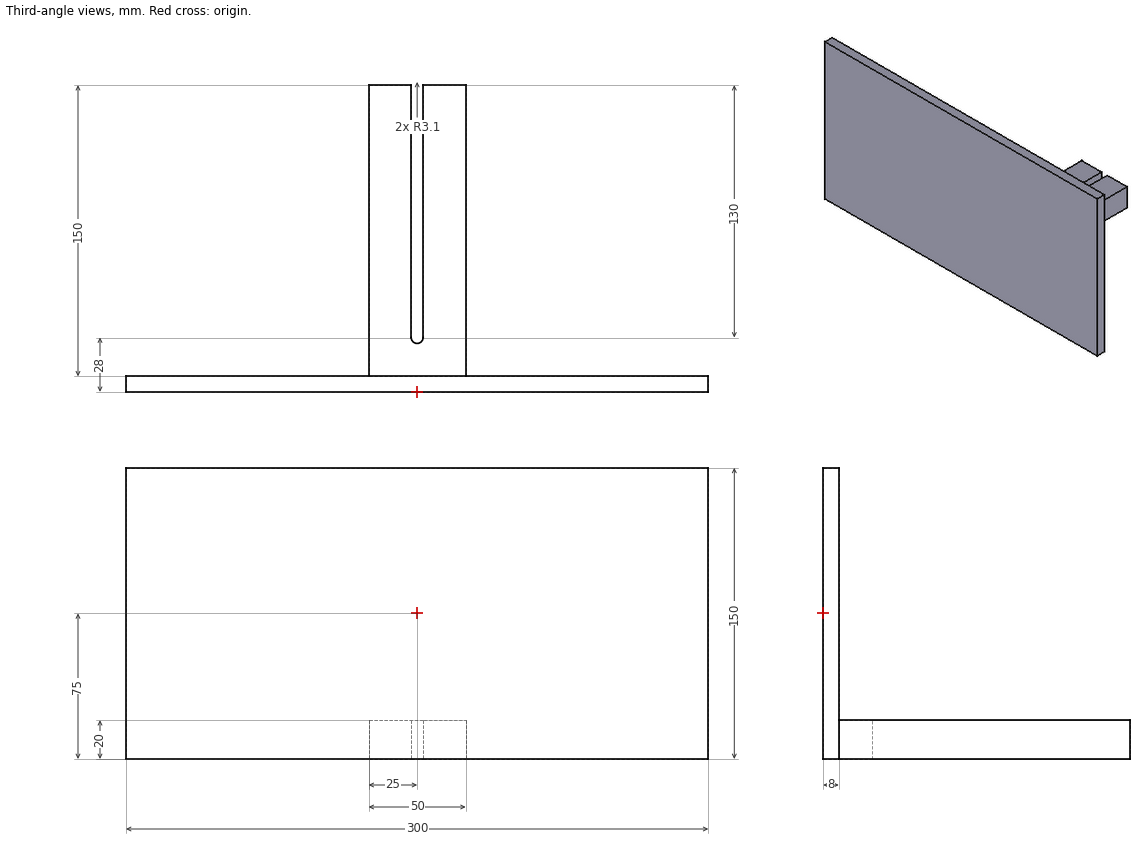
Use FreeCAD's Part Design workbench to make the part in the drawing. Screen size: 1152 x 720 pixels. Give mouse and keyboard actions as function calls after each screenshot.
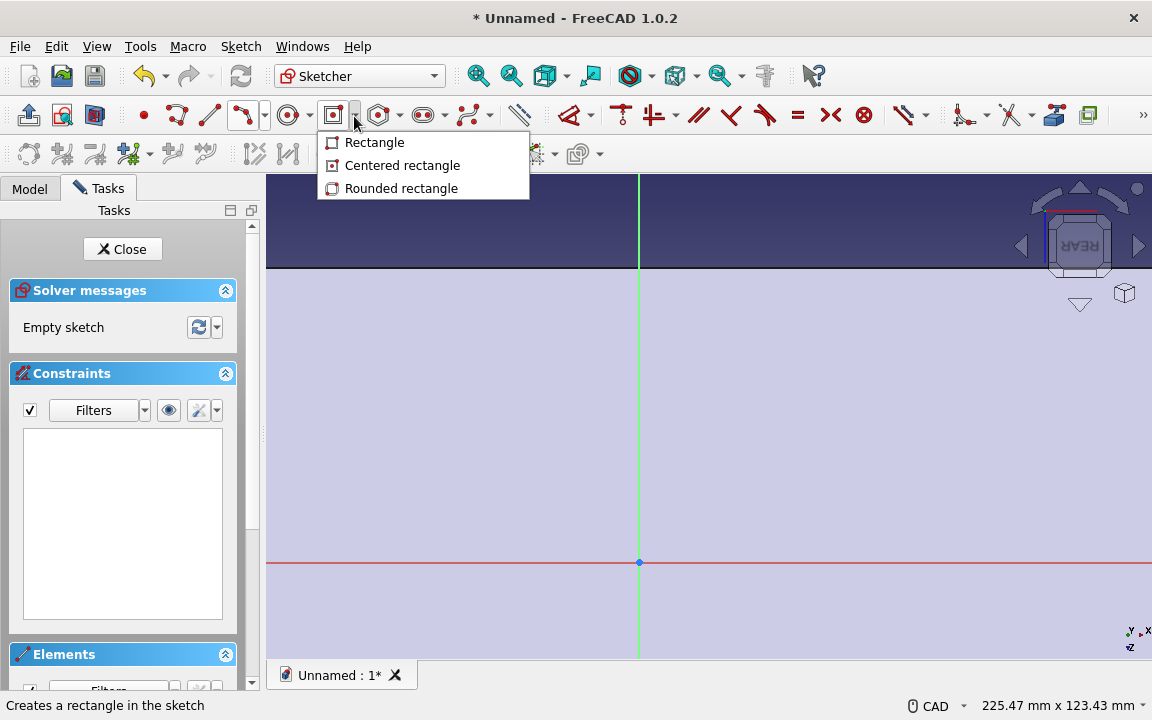
click(424, 142)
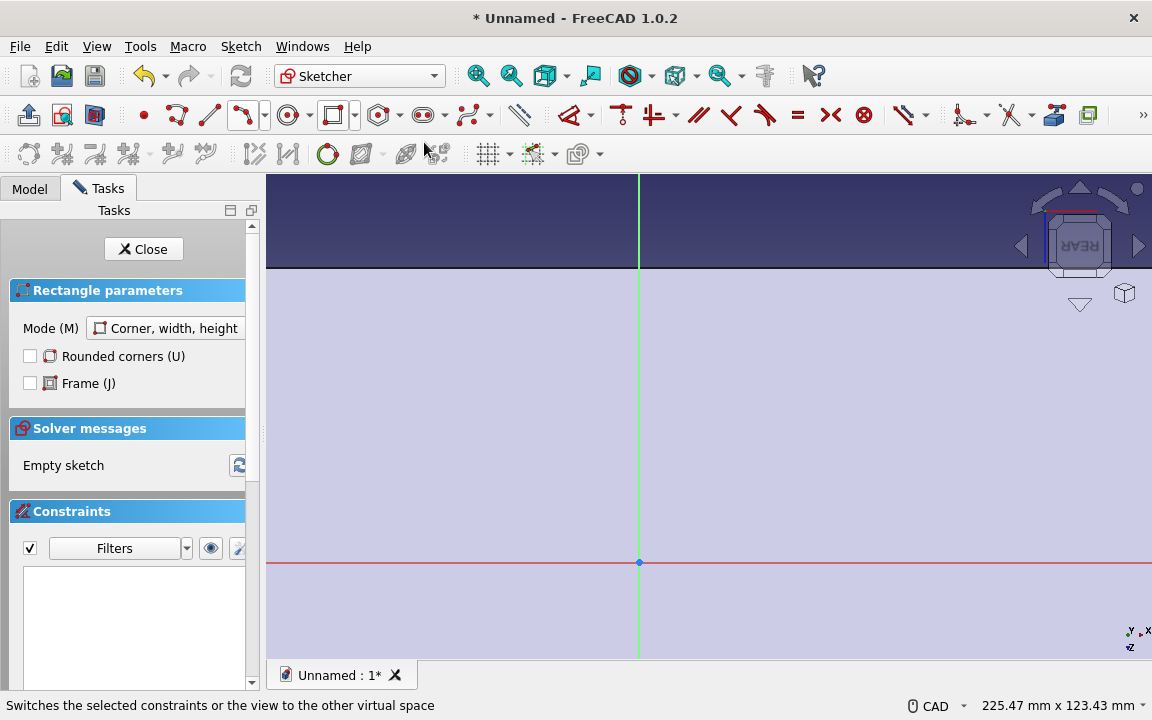
click(541, 268)
click(738, 347)
key(Escape)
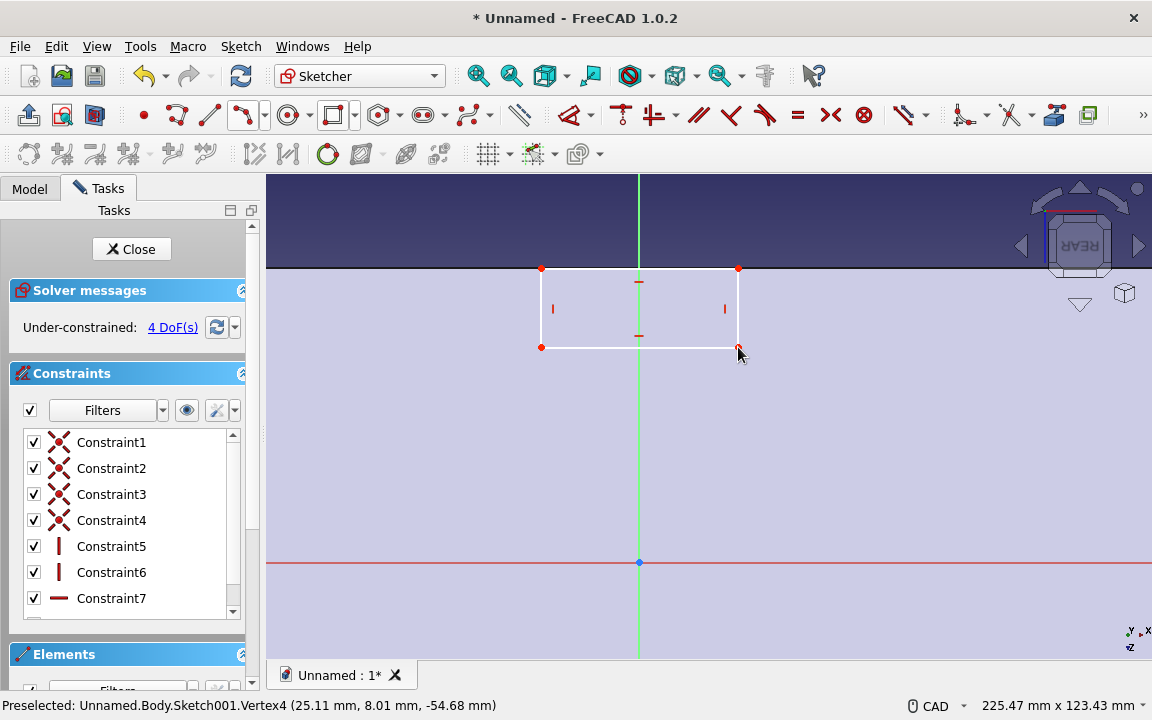
click(568, 116)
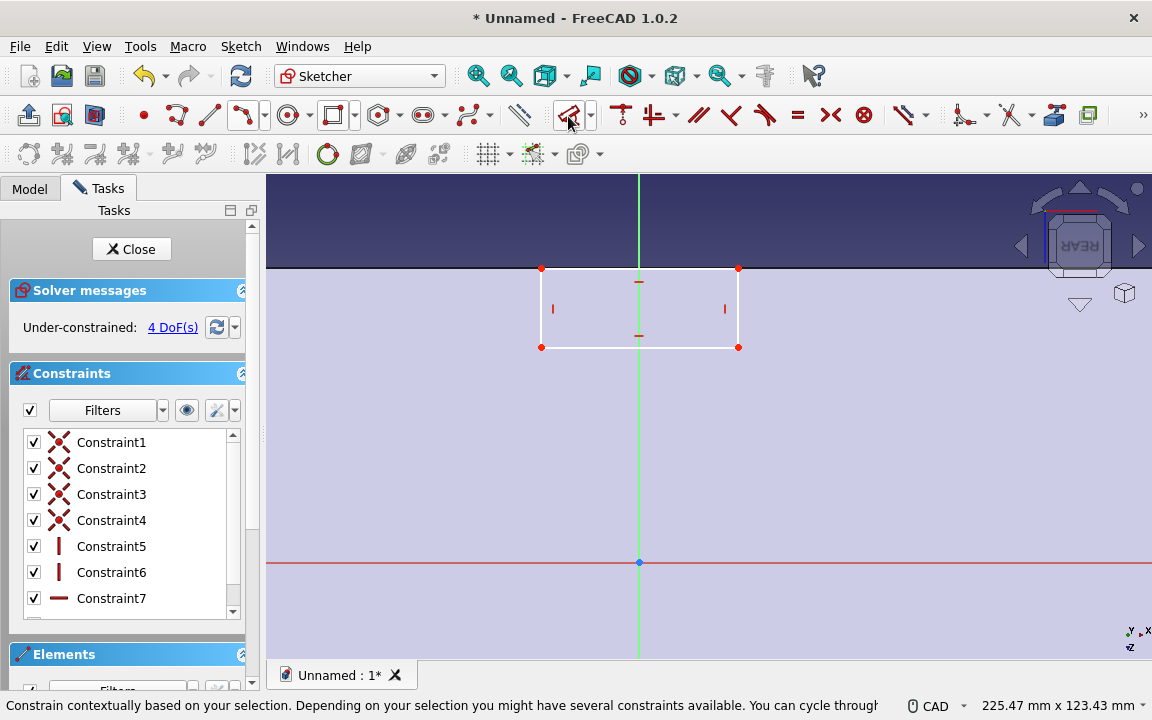
click(541, 293)
click(507, 308)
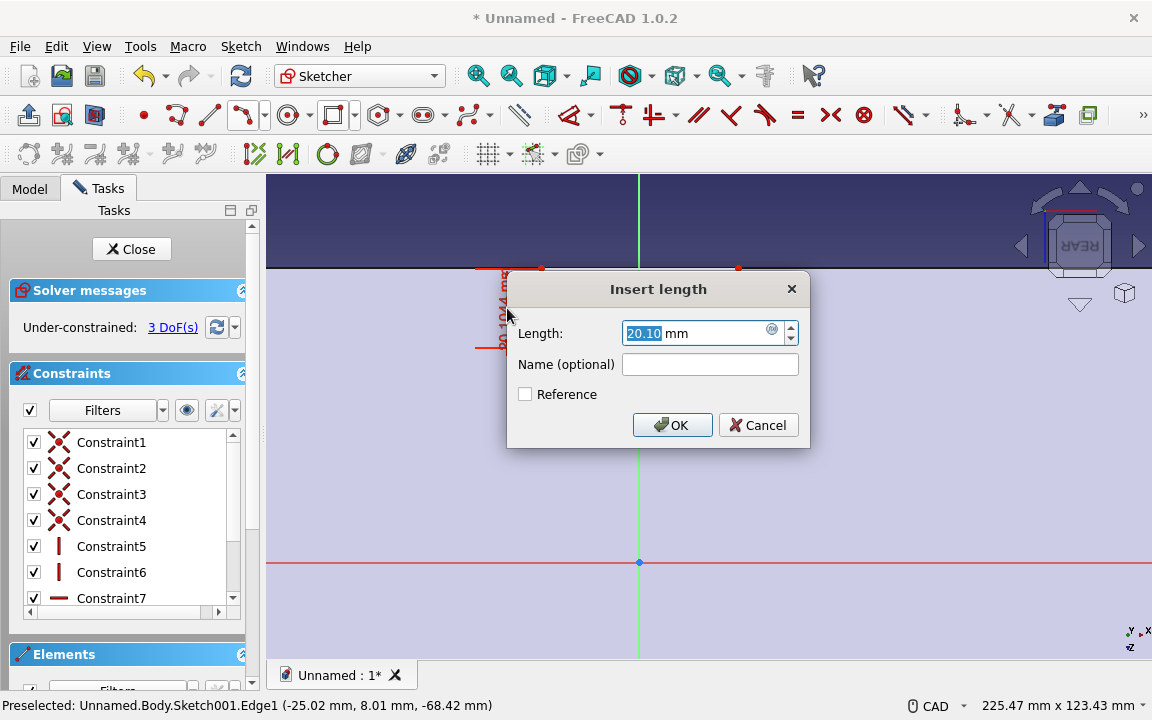
text(20)
key(Return)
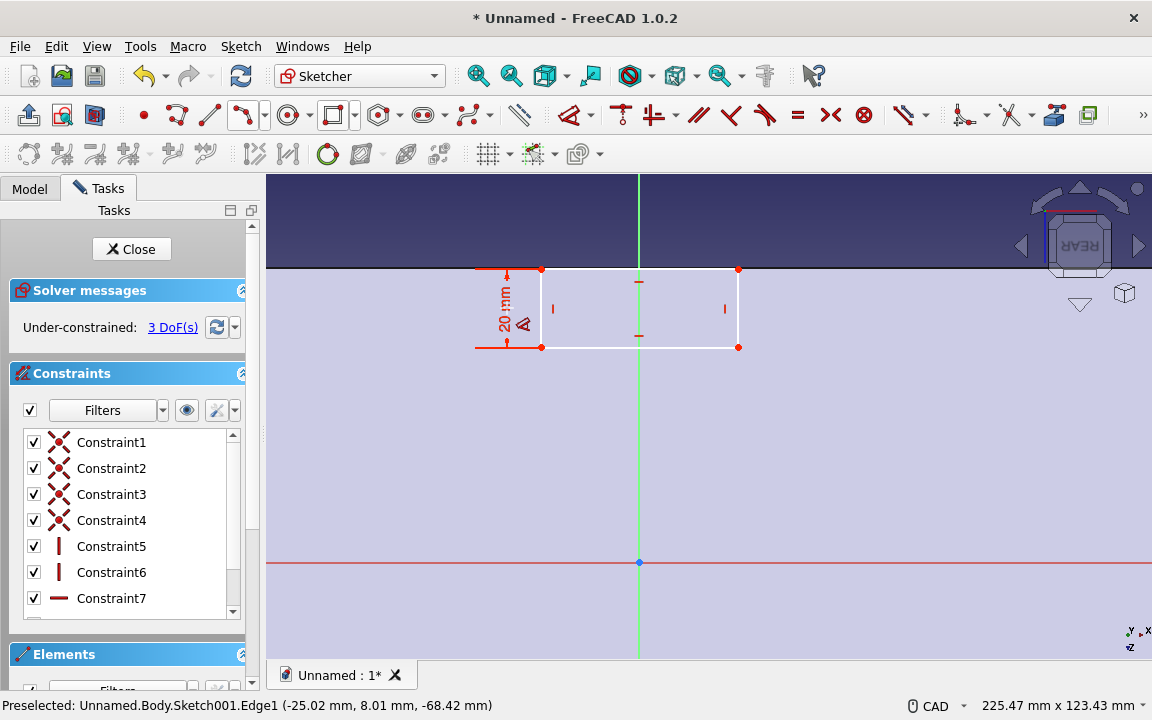
click(600, 348)
click(594, 314)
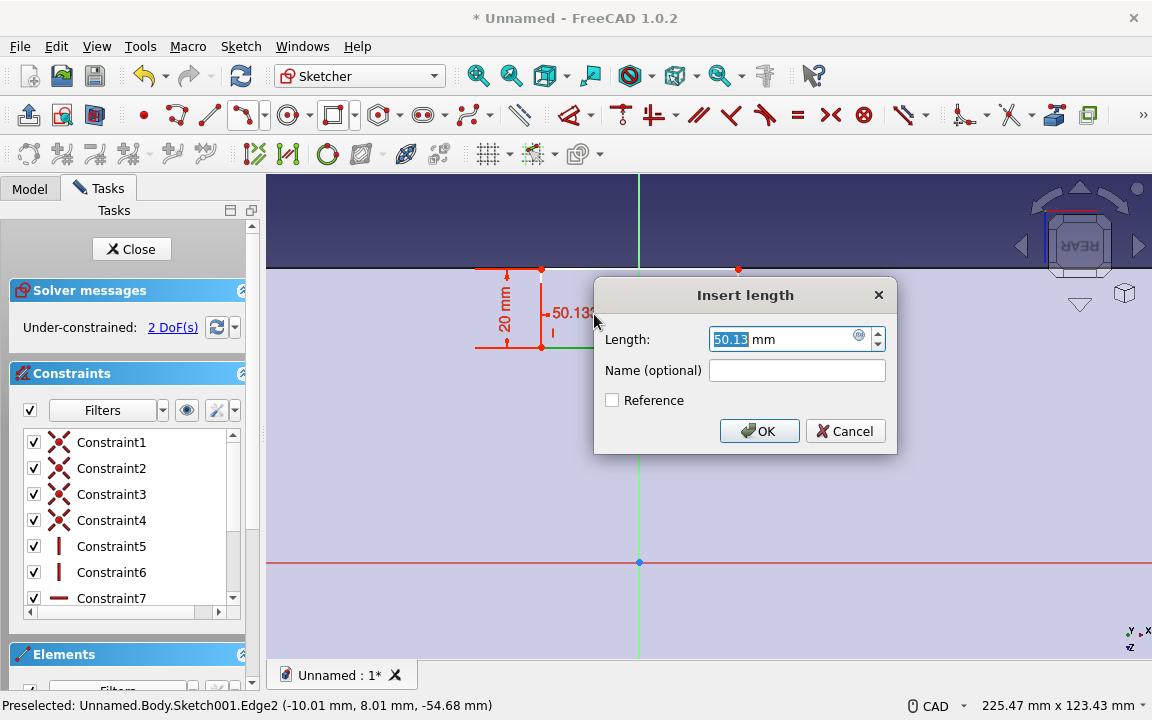
text(50)
key(Return)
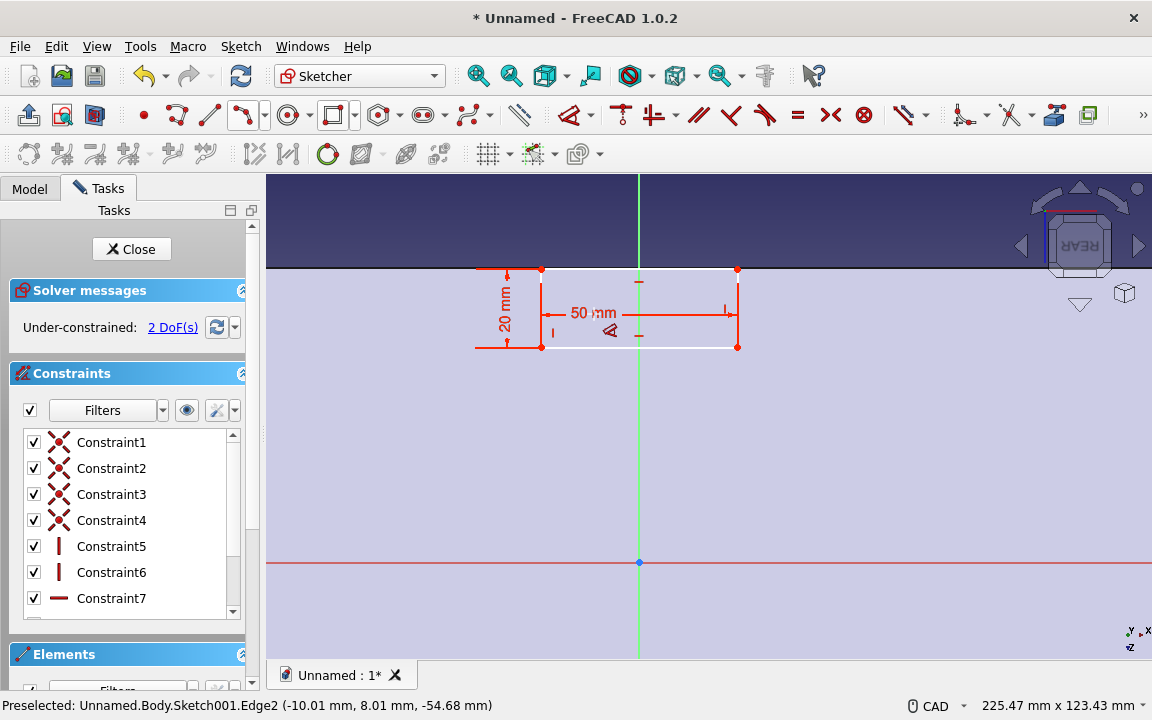
click(541, 269)
click(590, 597)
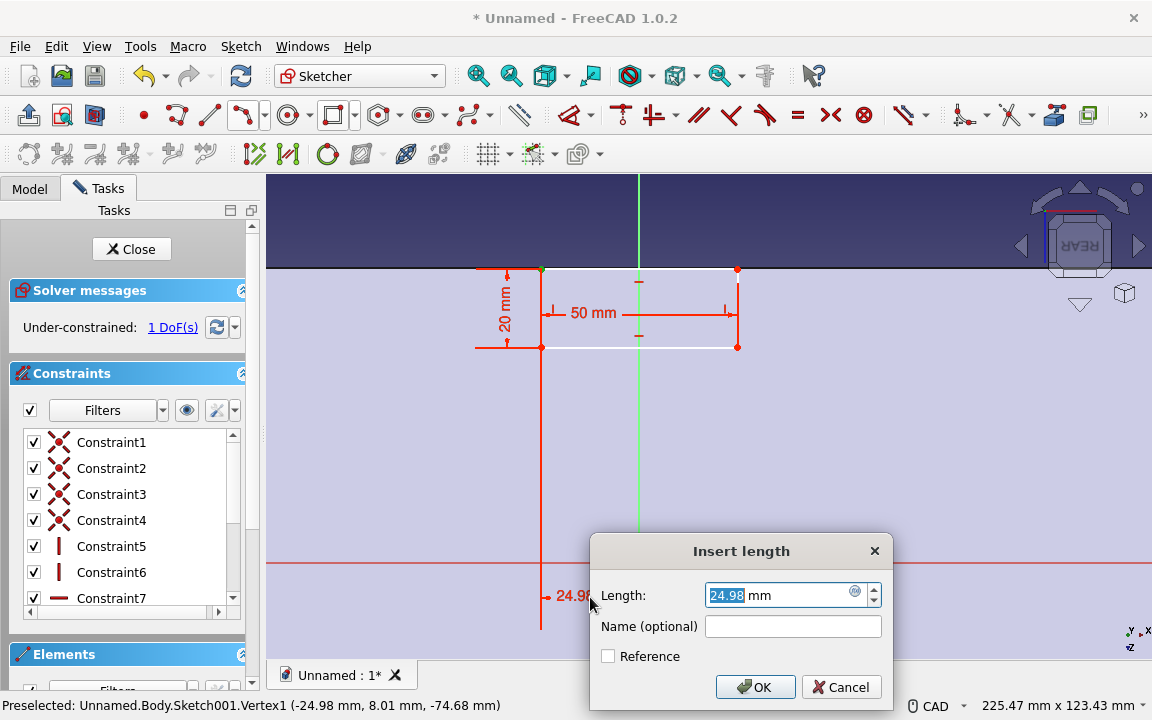
text(25)
key(Return)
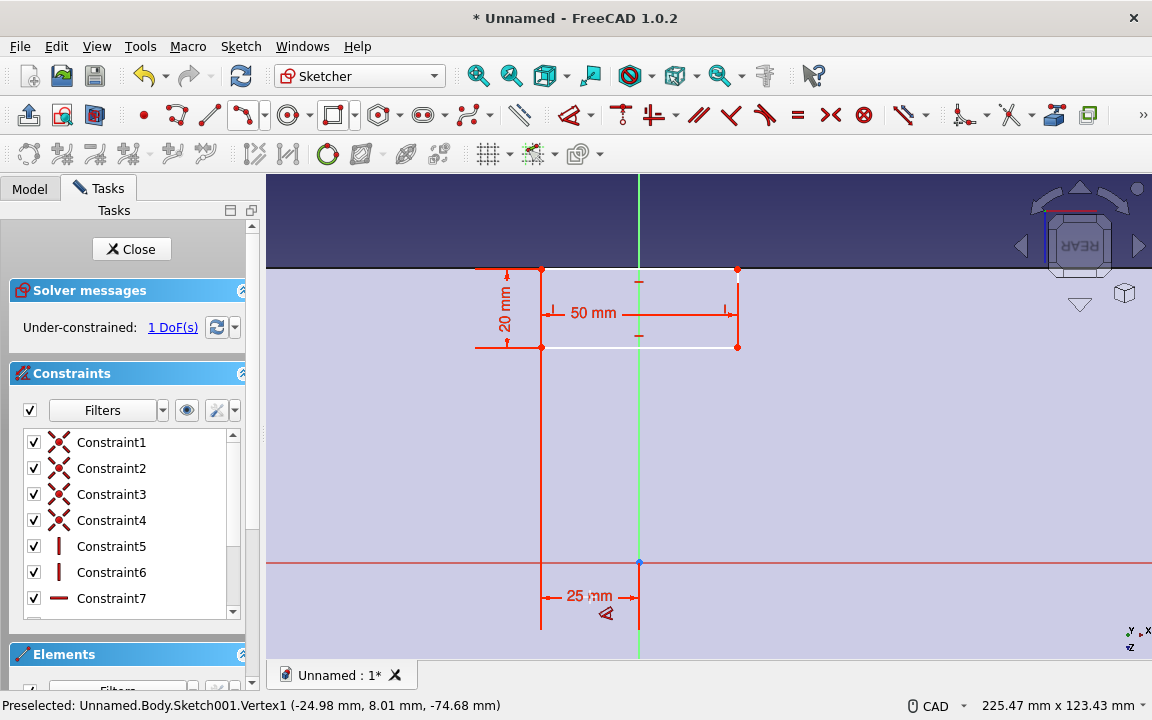
click(541, 269)
click(507, 416)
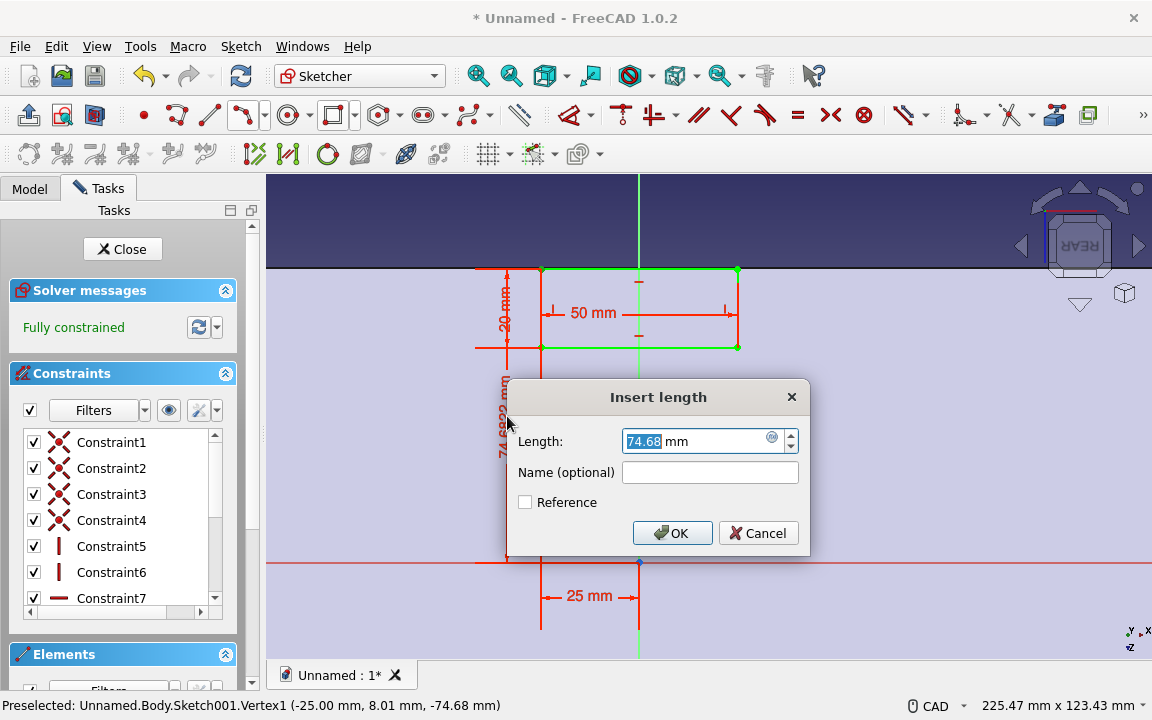
text(75)
key(Return)
key(Escape)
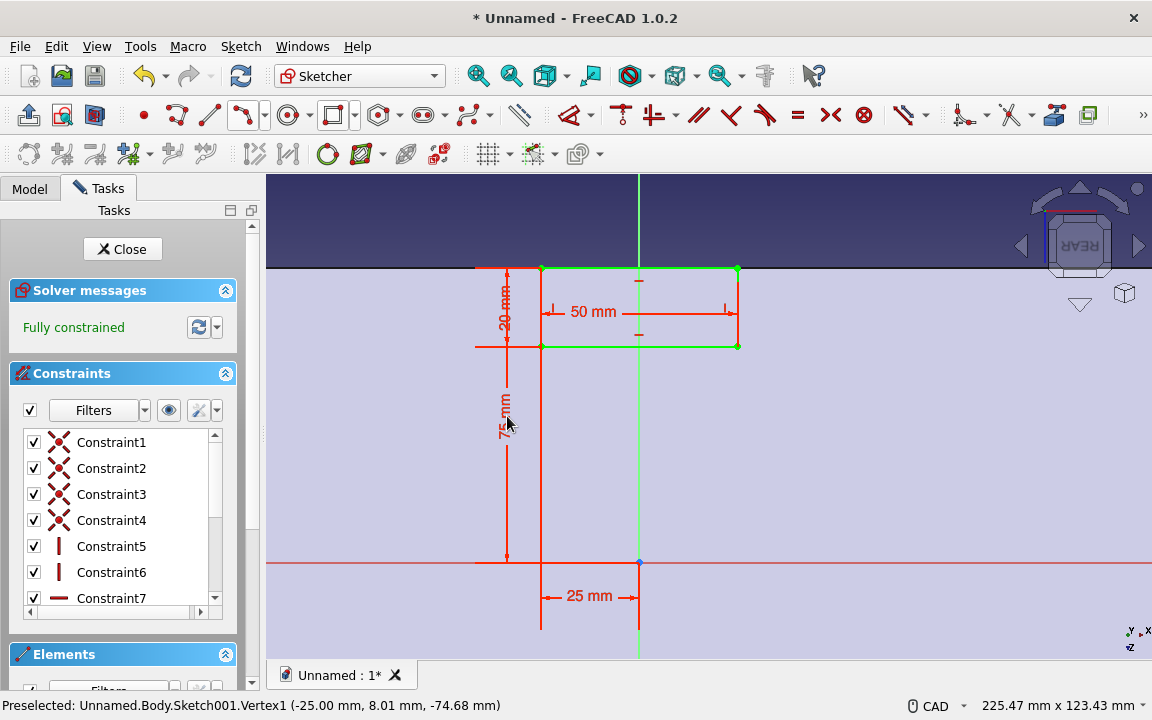
click(123, 249)